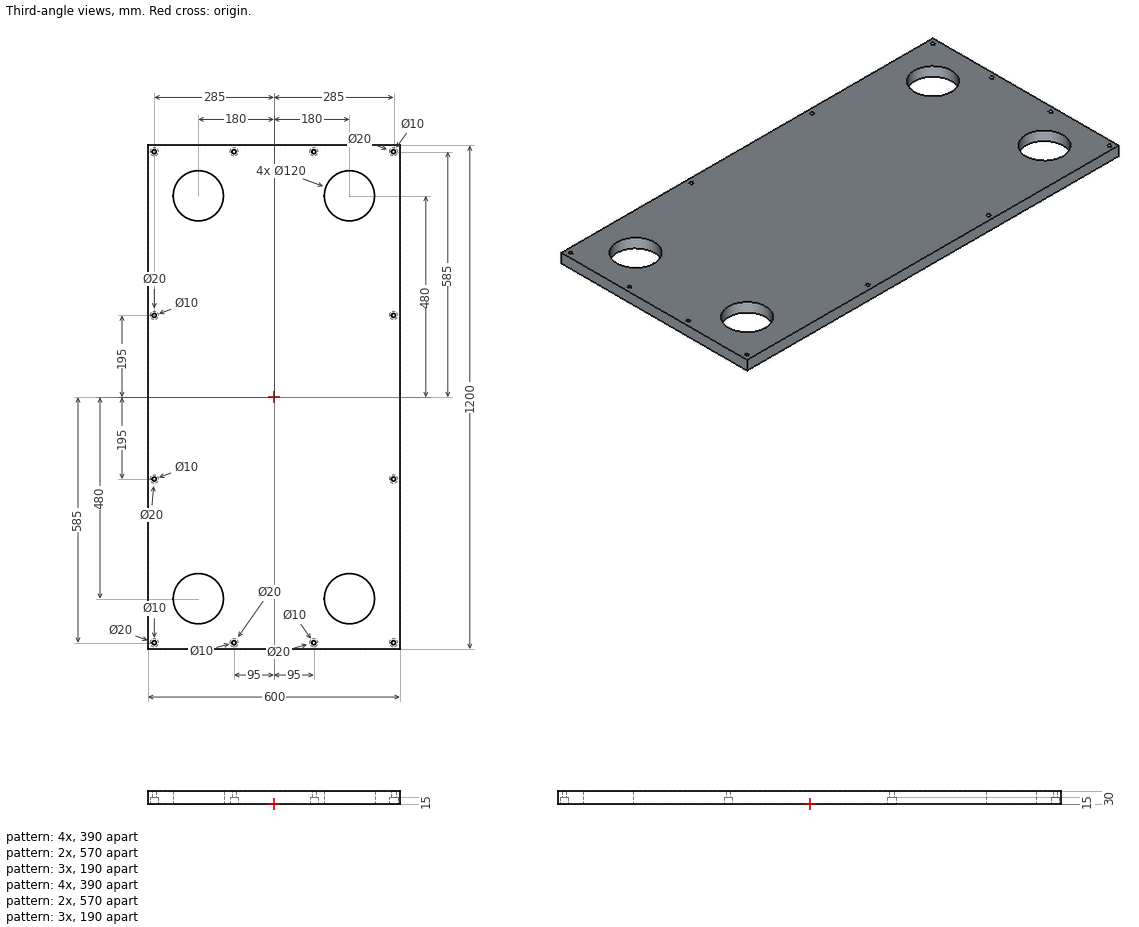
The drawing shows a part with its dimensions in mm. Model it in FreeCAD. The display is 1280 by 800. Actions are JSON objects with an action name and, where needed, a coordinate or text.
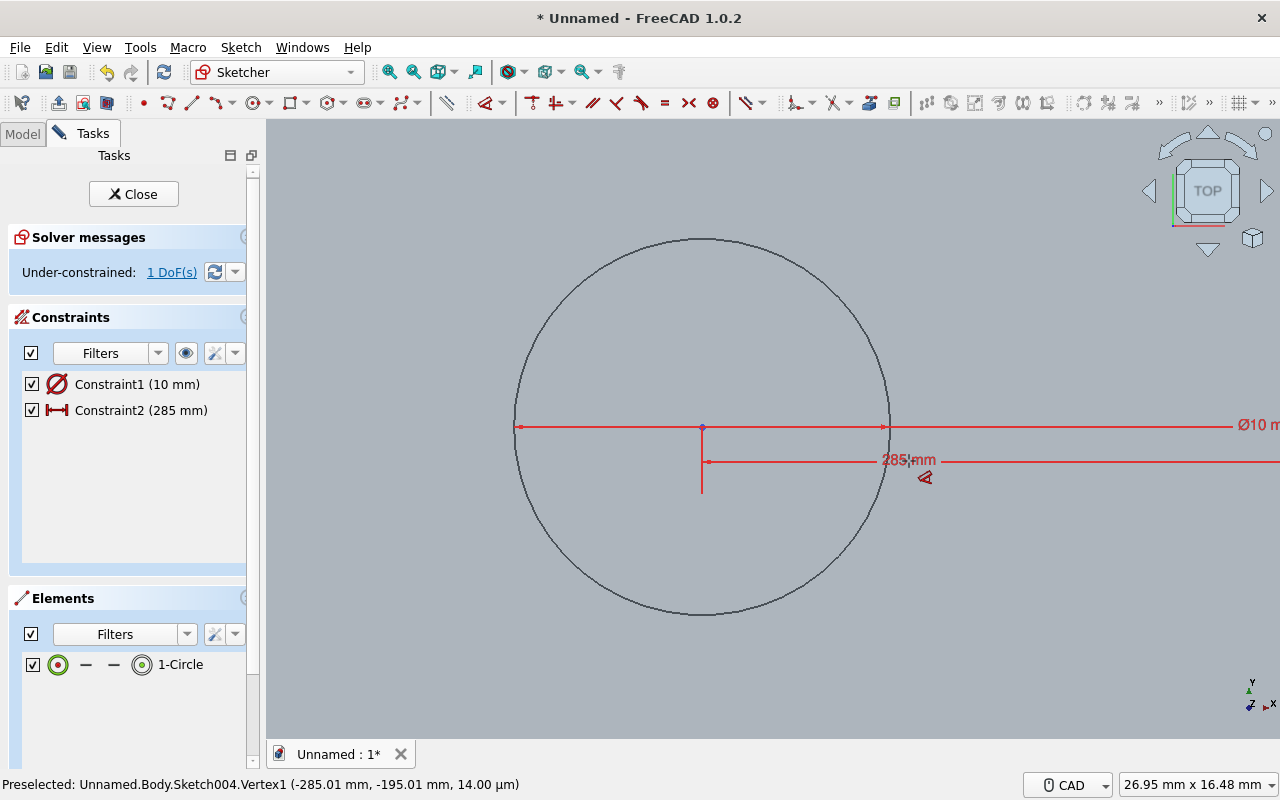
{"action": "left_click", "coordinate": [702, 427]}
{"action": "left_click", "coordinate": [668, 287]}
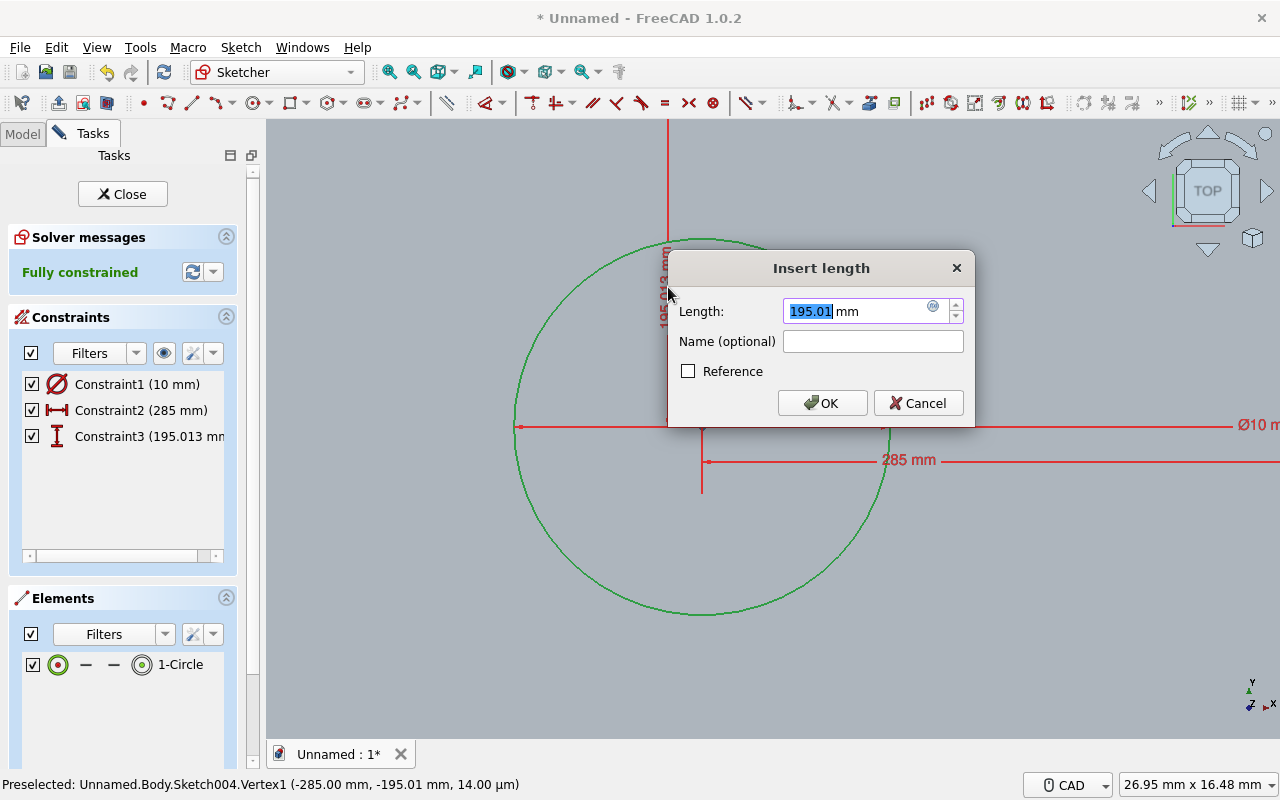
{"action": "type", "text": "195"}
{"action": "key", "text": "Return"}
{"action": "key", "text": "Escape"}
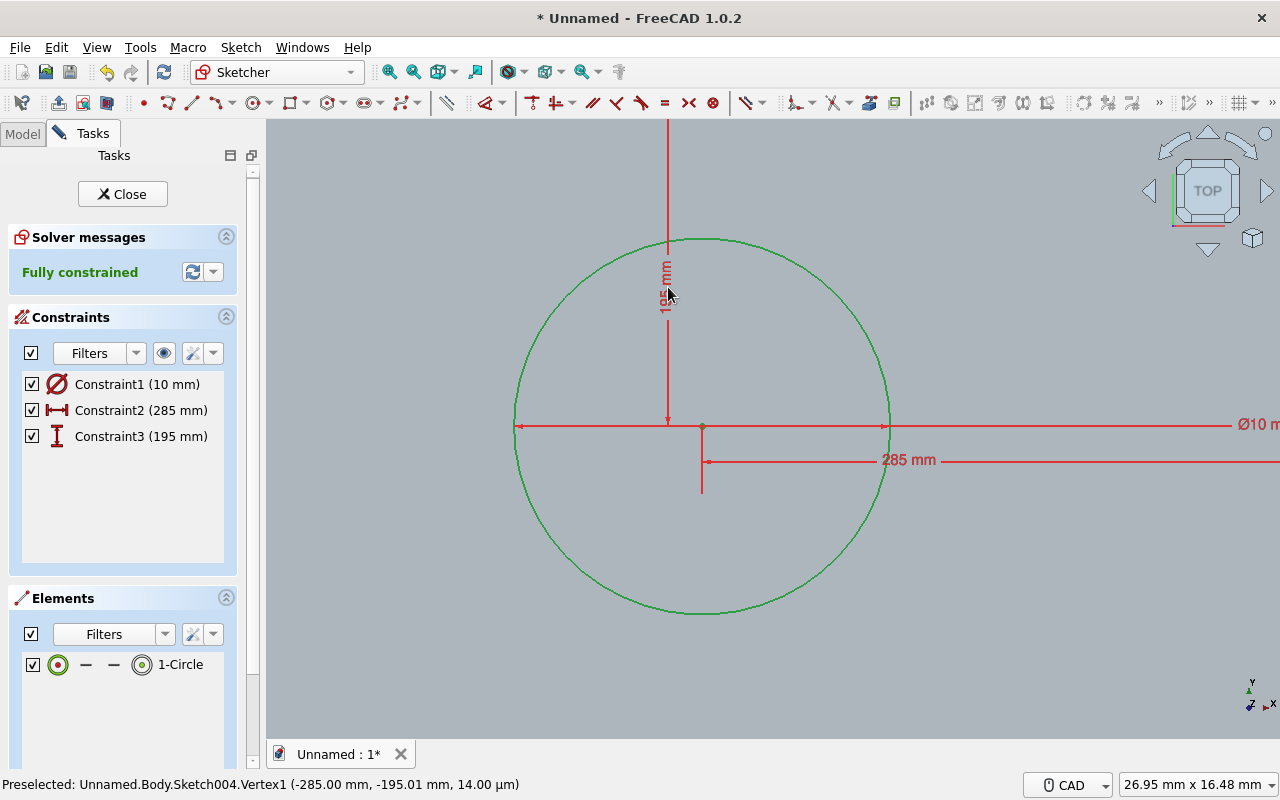
{"action": "left_click", "coordinate": [123, 194]}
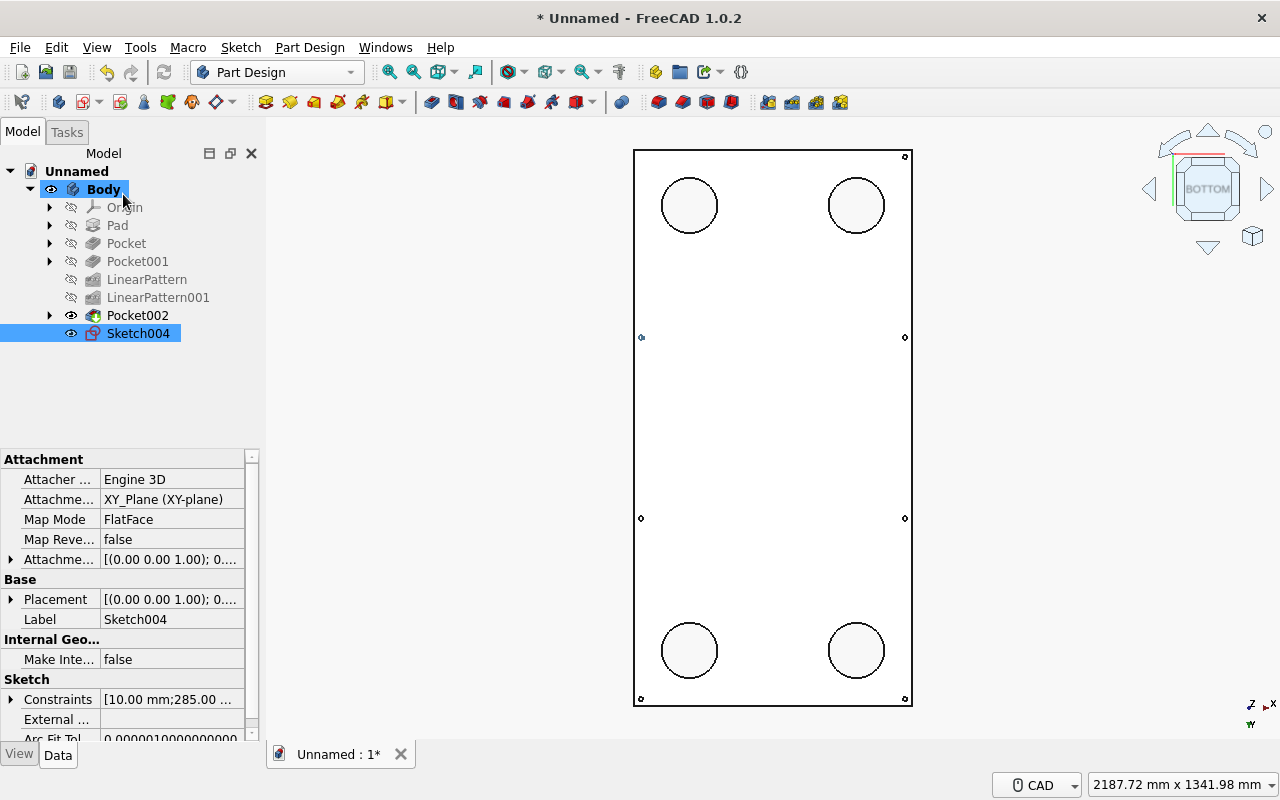
{"action": "left_click", "coordinate": [432, 102]}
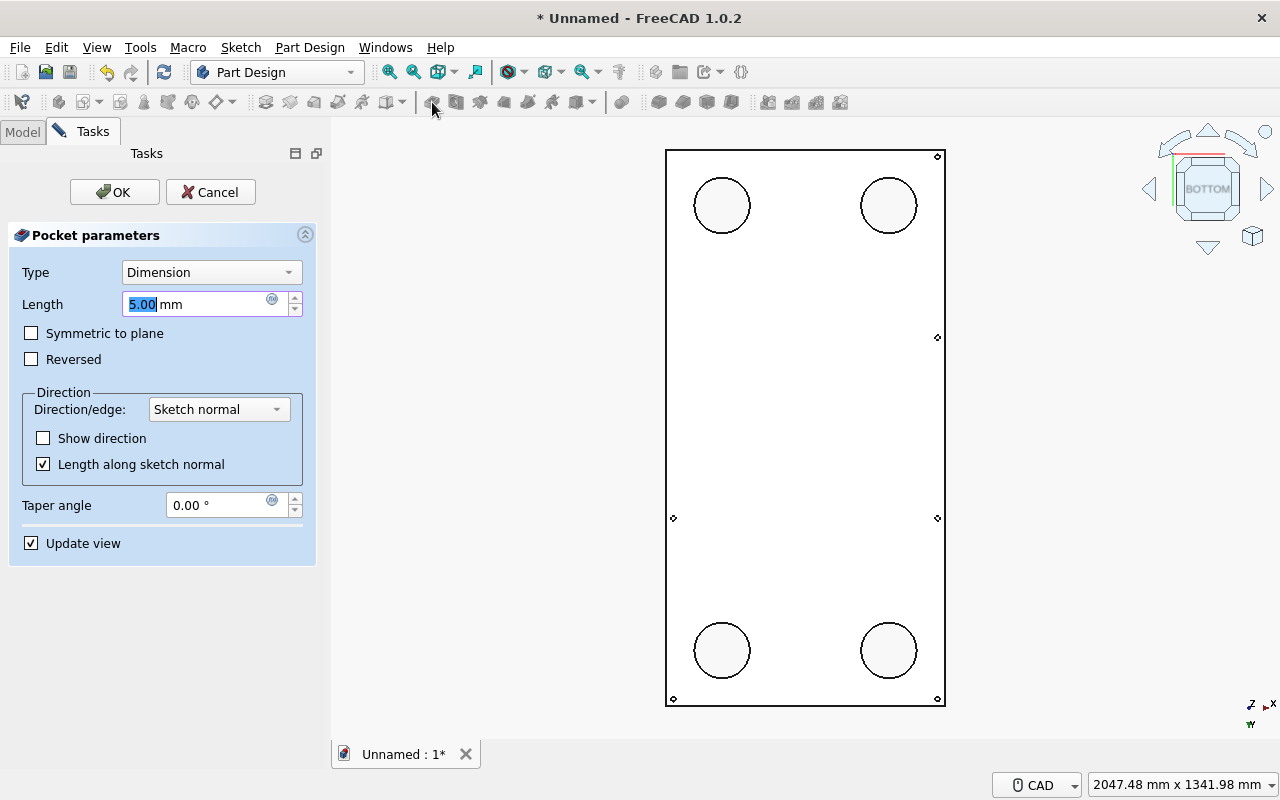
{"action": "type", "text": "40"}
{"action": "key", "text": "Tab"}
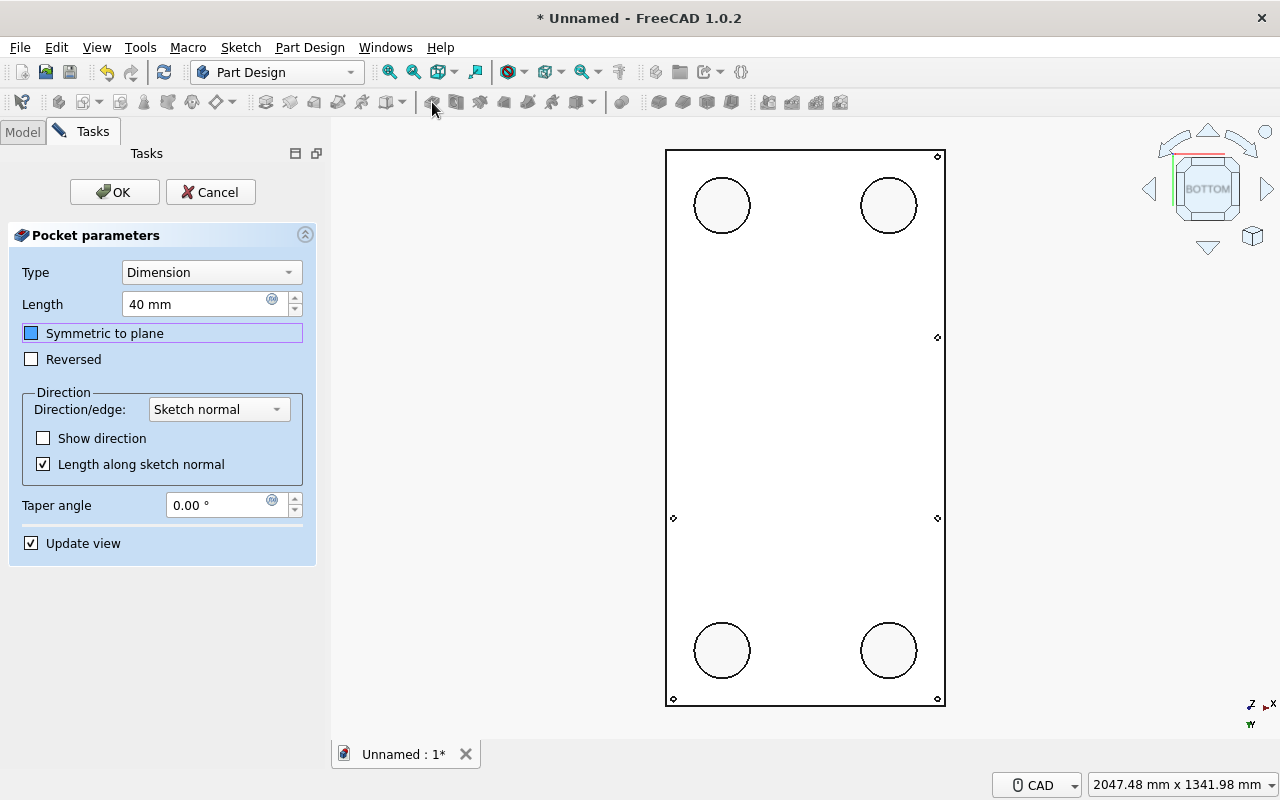
{"action": "left_click", "coordinate": [30, 359]}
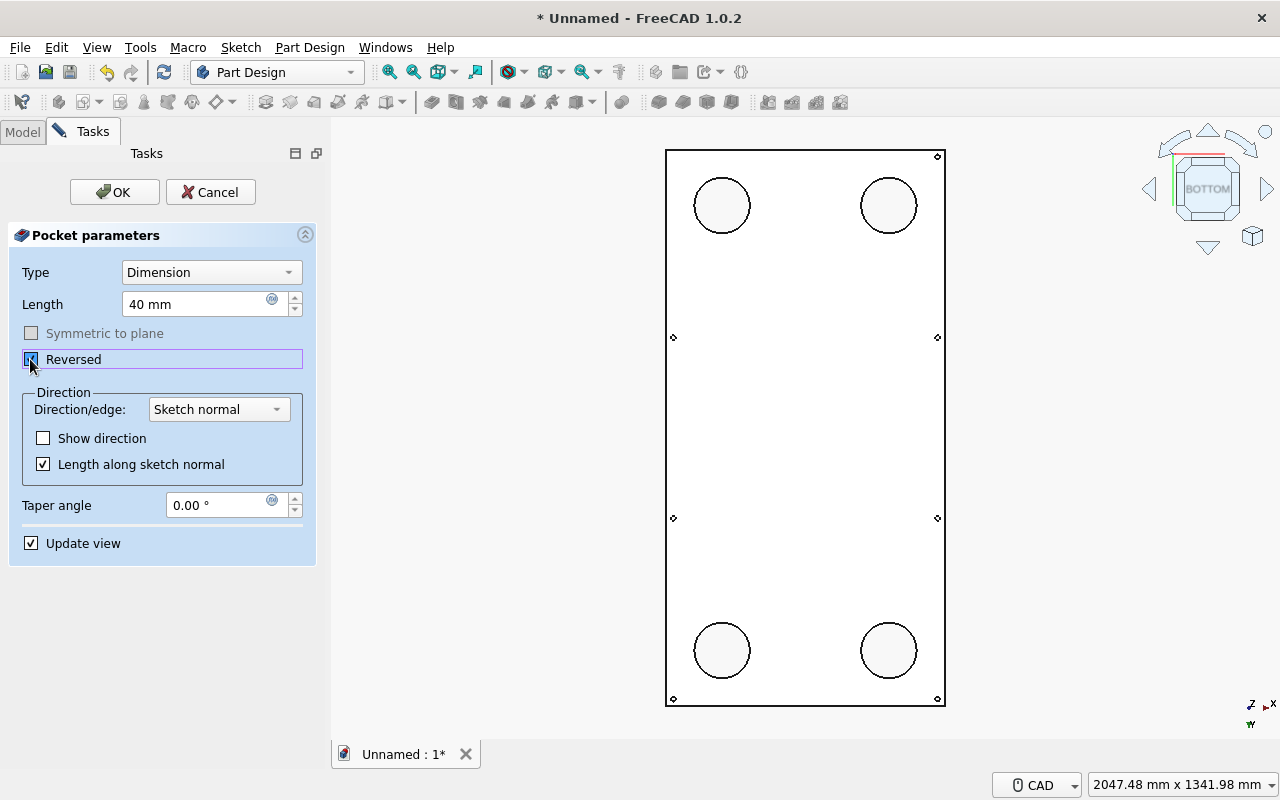
{"action": "left_click", "coordinate": [115, 192]}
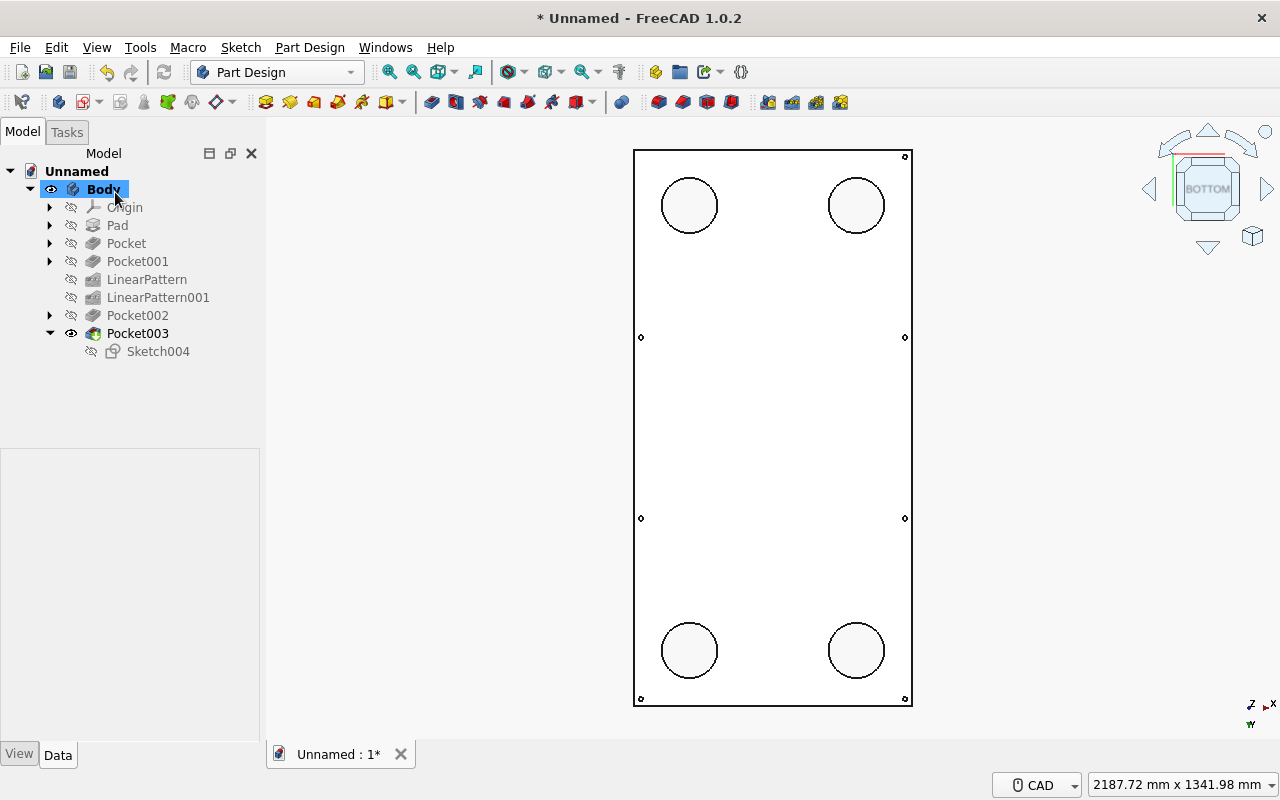
{"action": "left_click", "coordinate": [773, 427]}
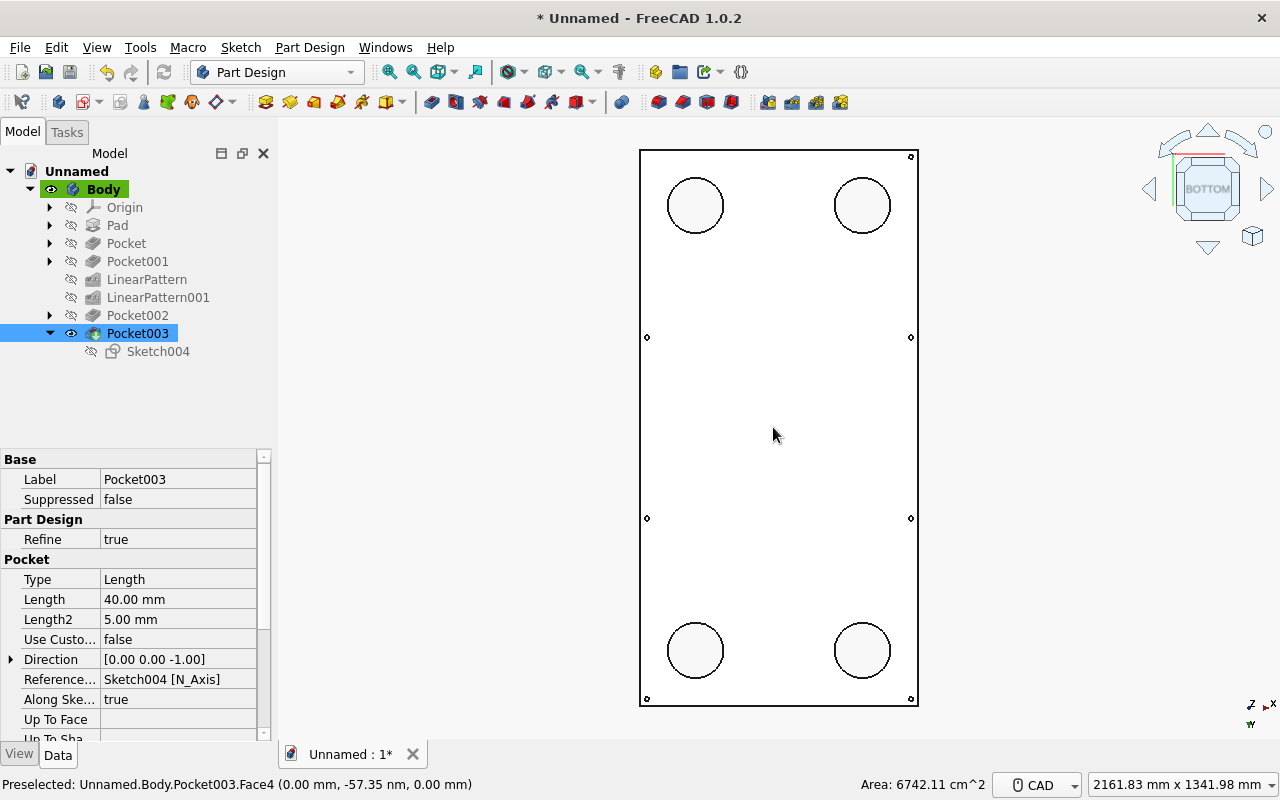
{"action": "left_click", "coordinate": [84, 102]}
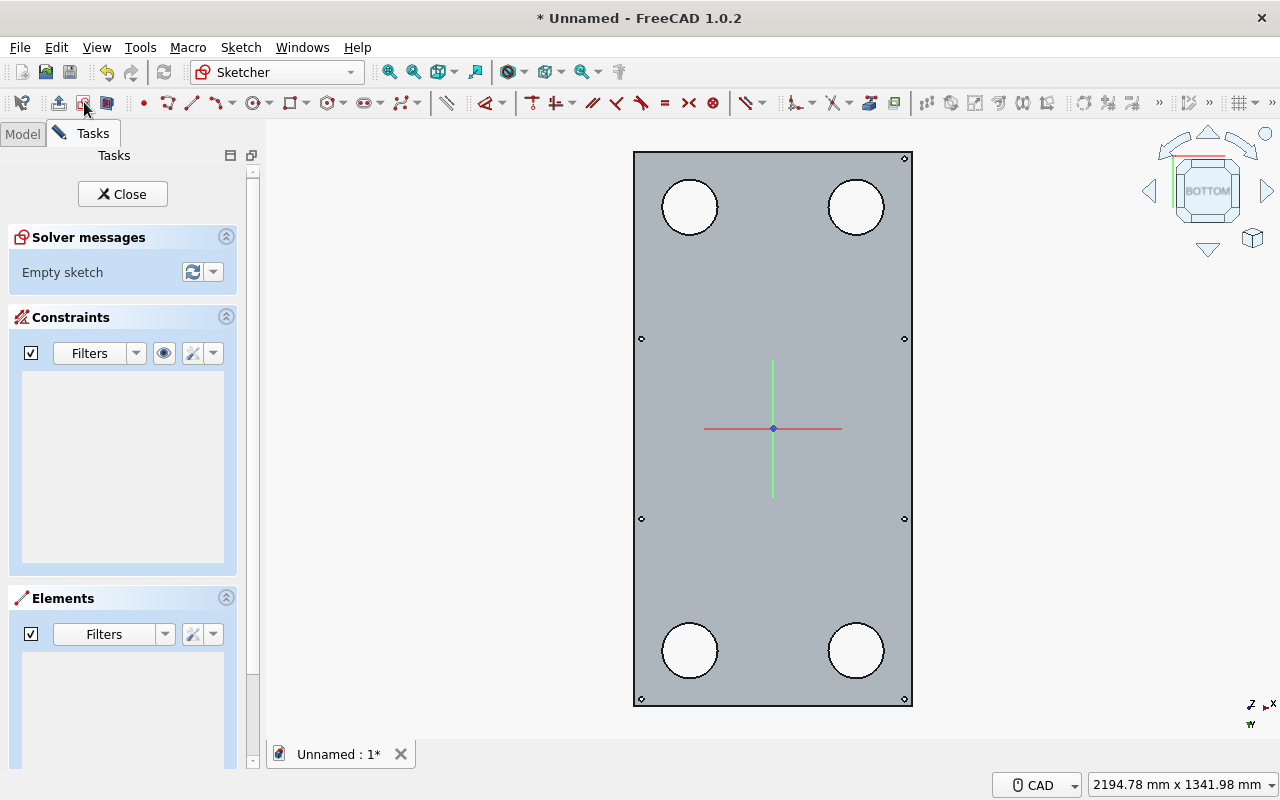
{"action": "scroll", "coordinate": [638, 147], "scroll_direction": "up", "scroll_amount": 15}